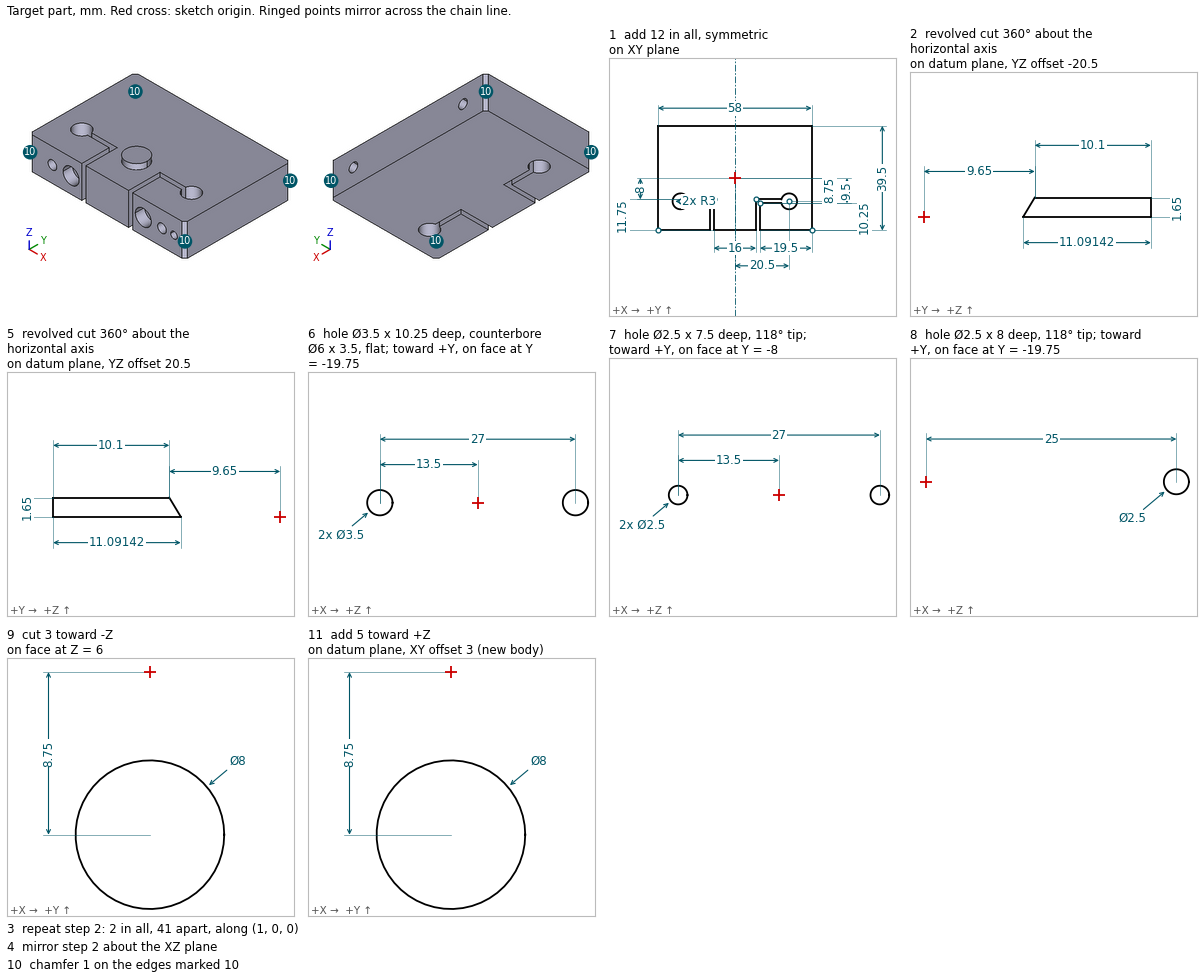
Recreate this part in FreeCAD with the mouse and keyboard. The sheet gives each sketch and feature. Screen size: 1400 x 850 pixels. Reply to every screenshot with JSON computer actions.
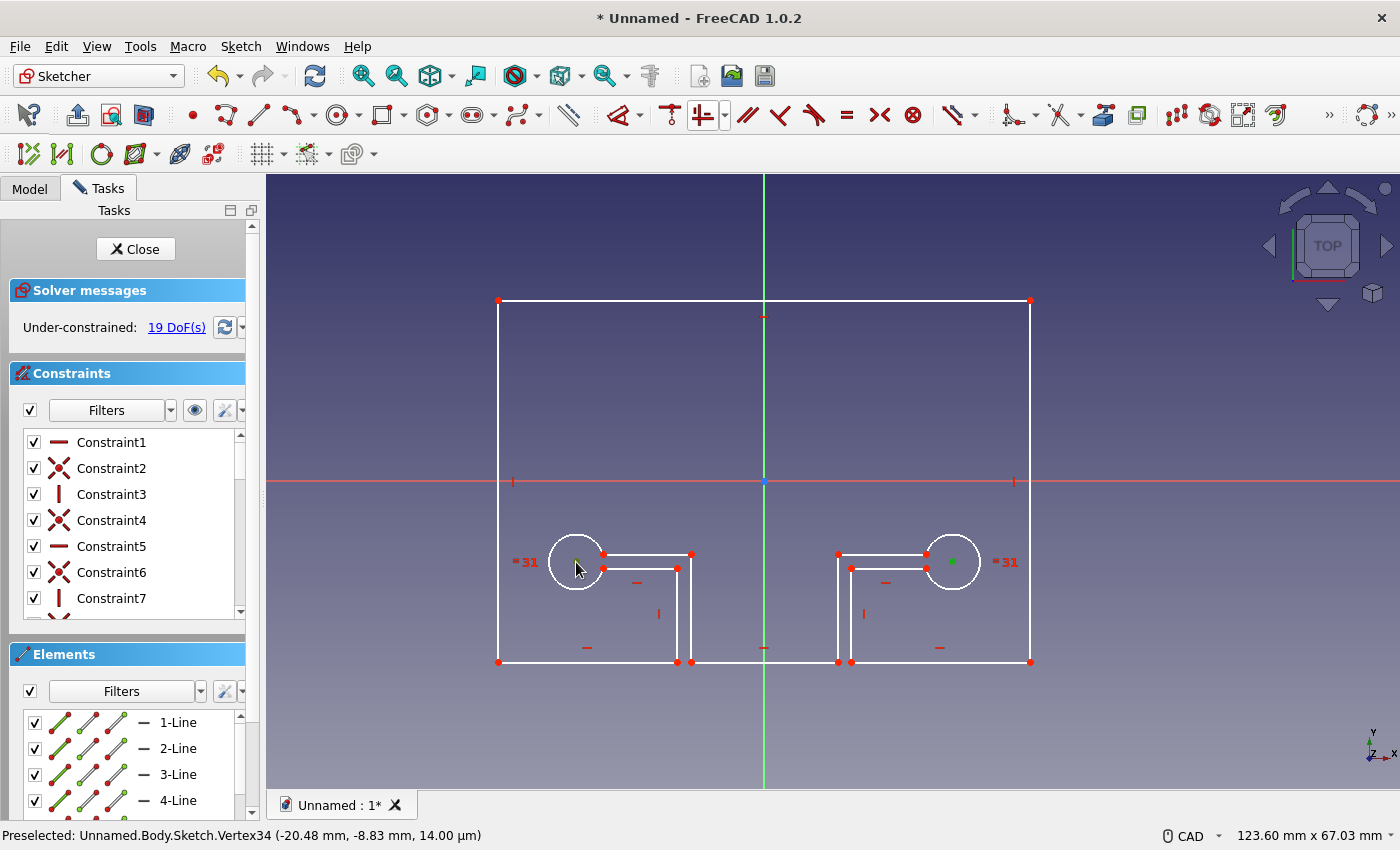
{"action": "left_click", "coordinate": [764, 721]}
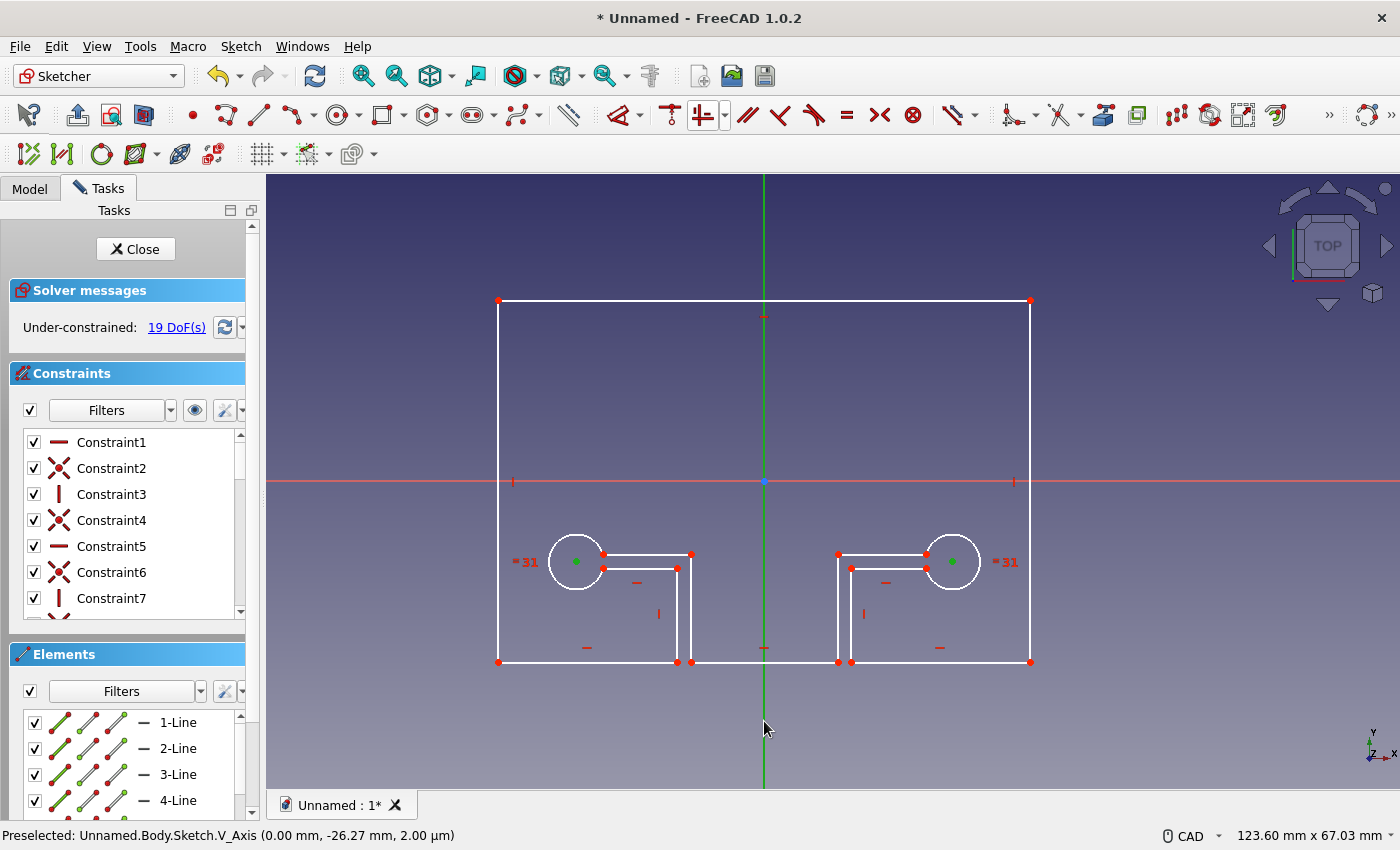
{"action": "left_click", "coordinate": [880, 116]}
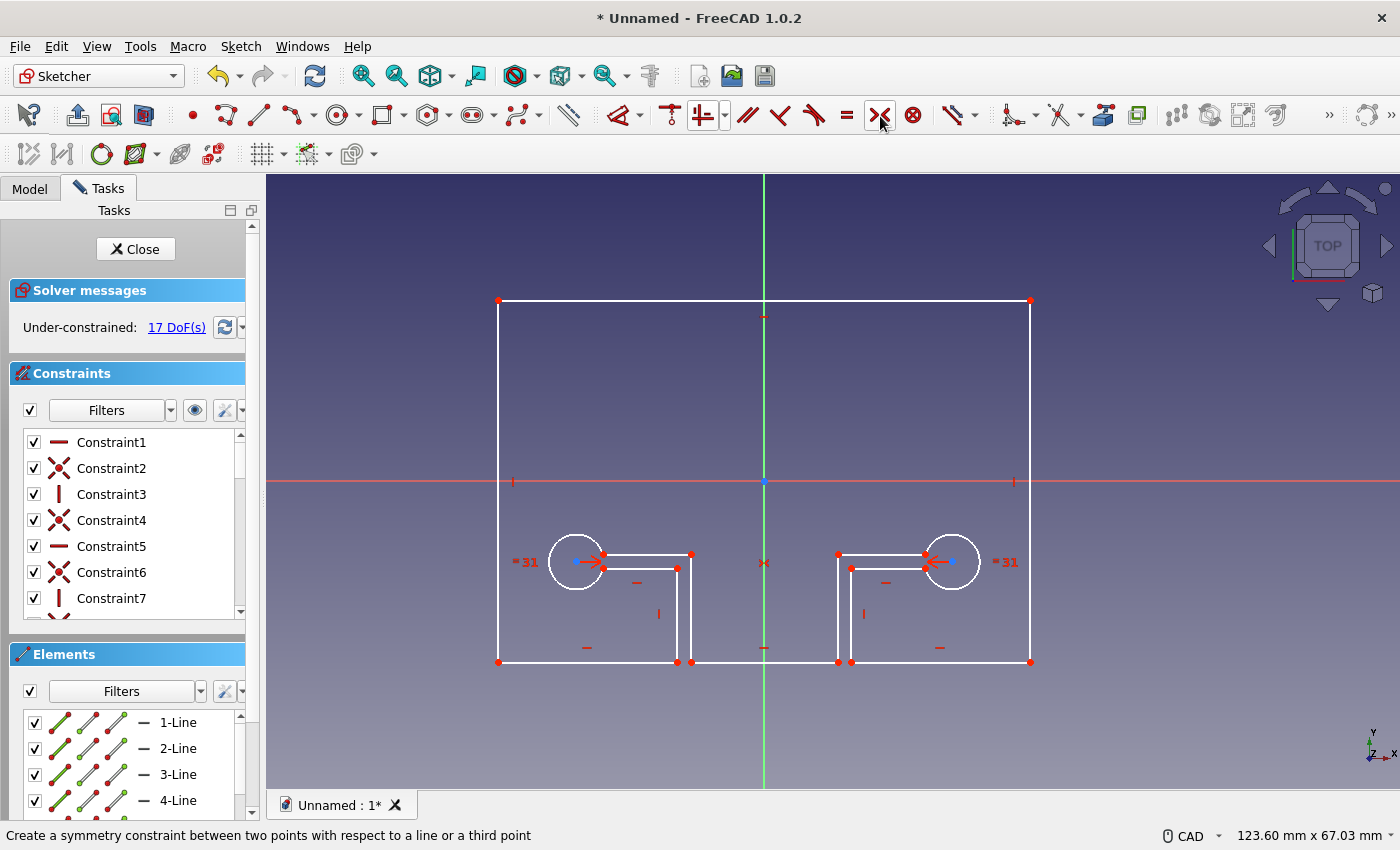
{"action": "left_click", "coordinate": [691, 555]}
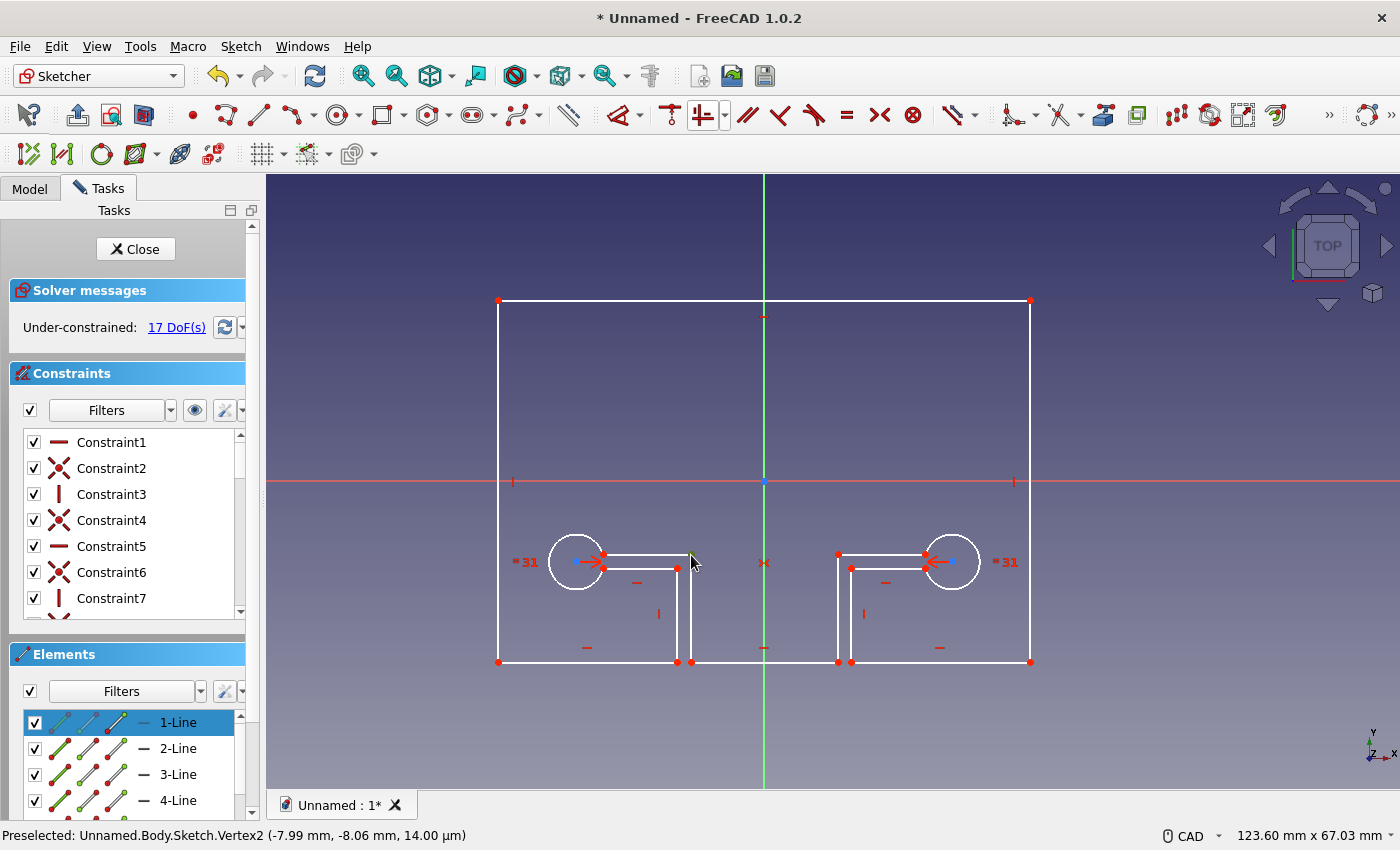
{"action": "left_click", "coordinate": [838, 555]}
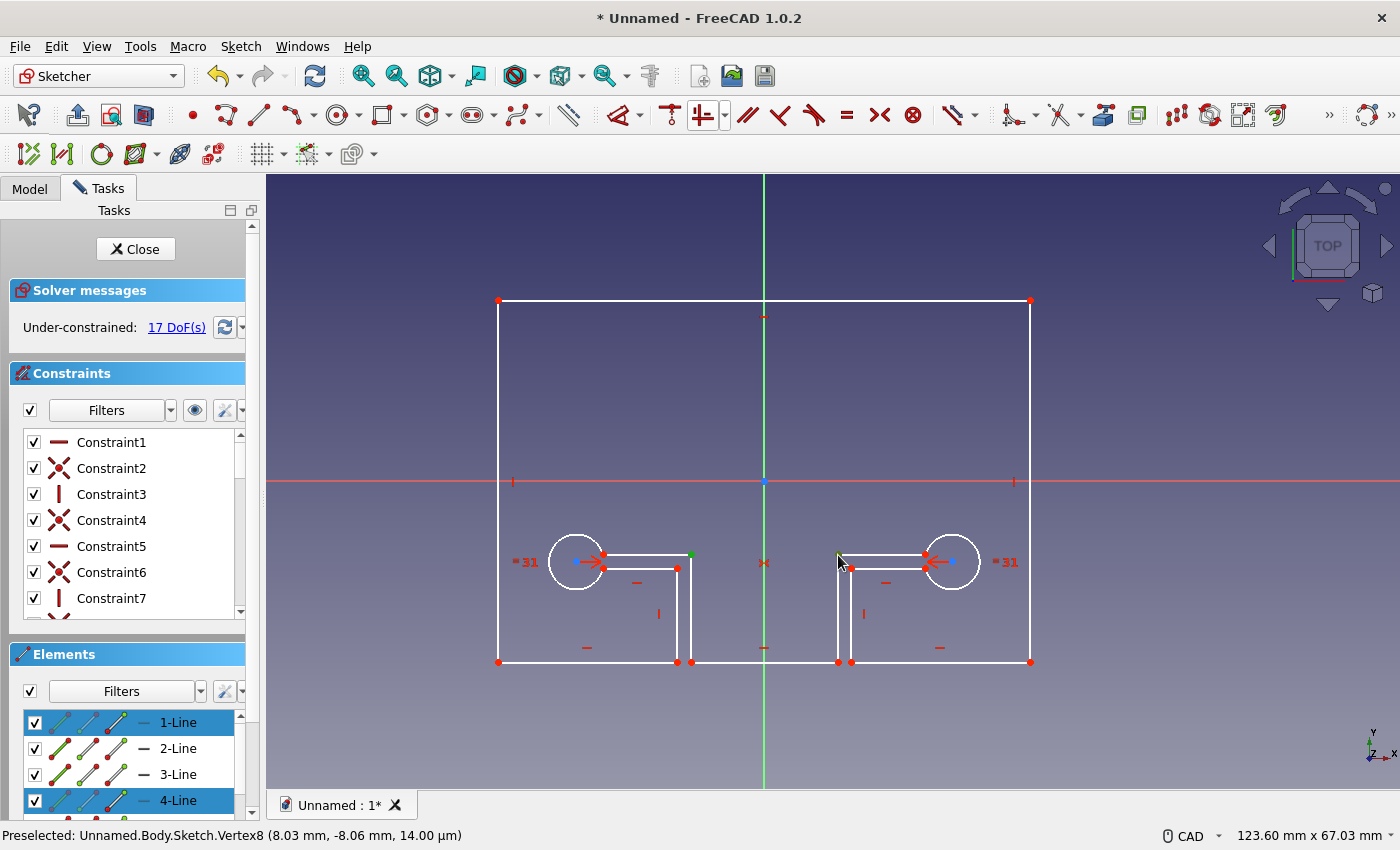
{"action": "left_click", "coordinate": [764, 721]}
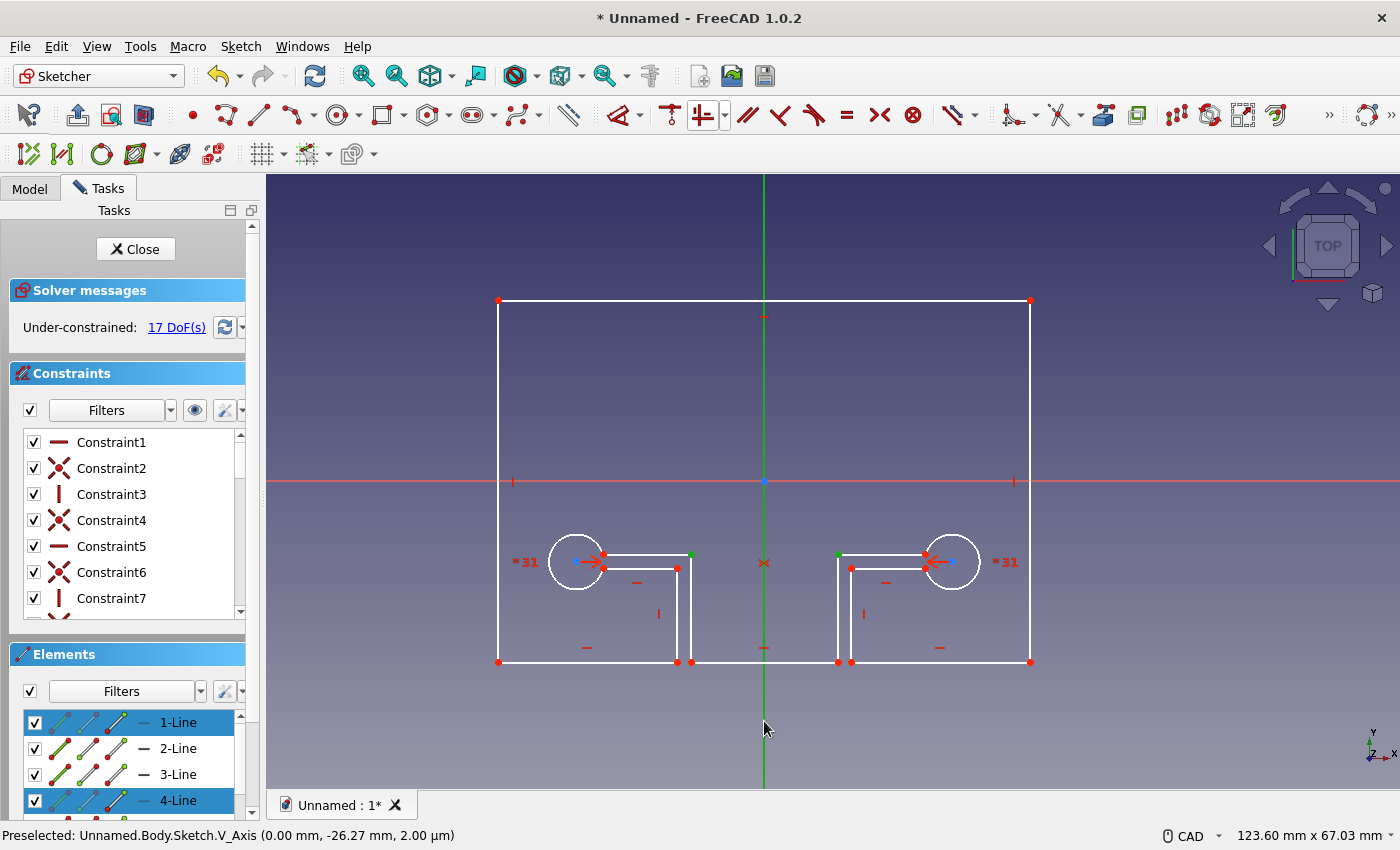
{"action": "left_click", "coordinate": [880, 116]}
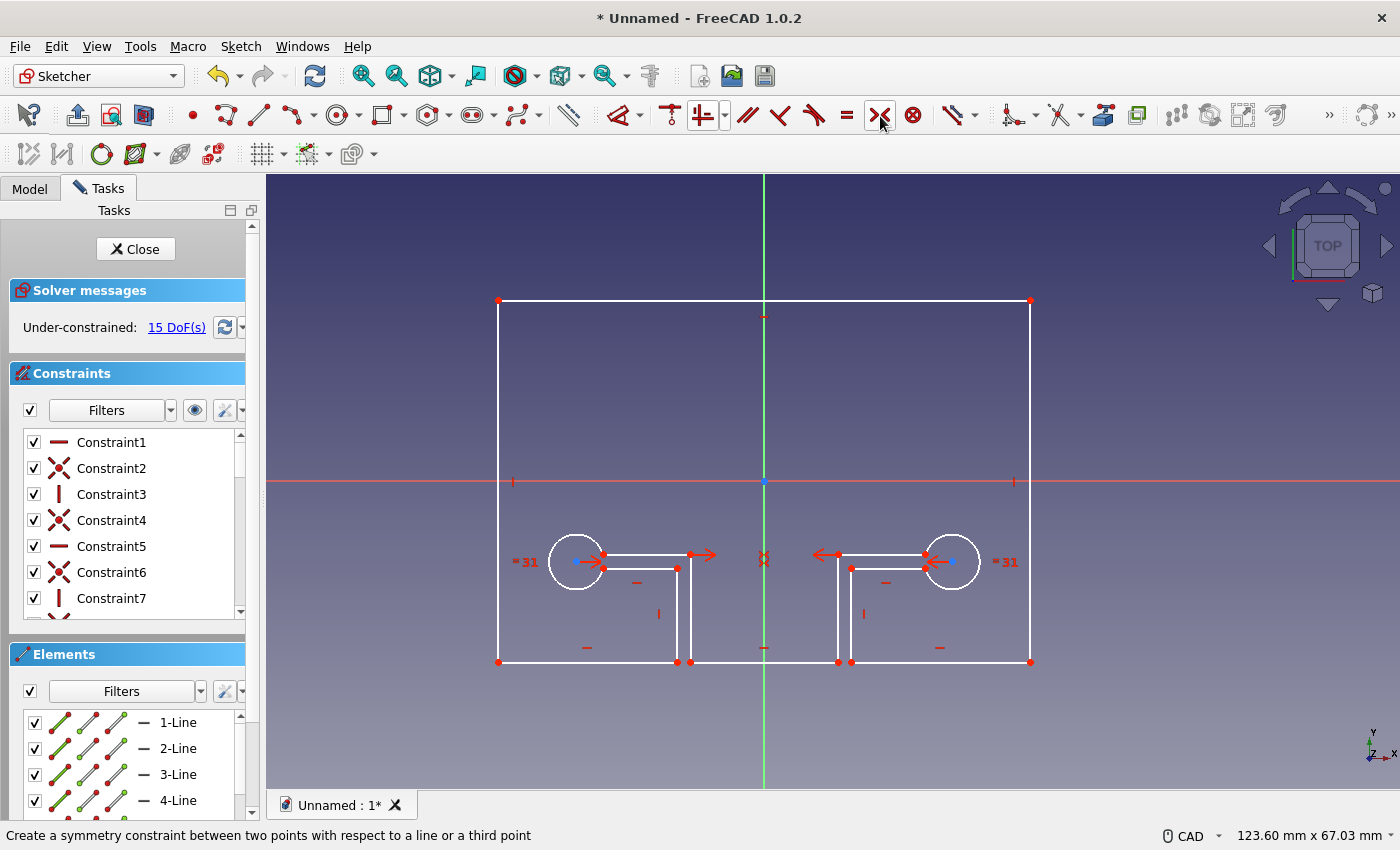
{"action": "left_click", "coordinate": [1030, 663]}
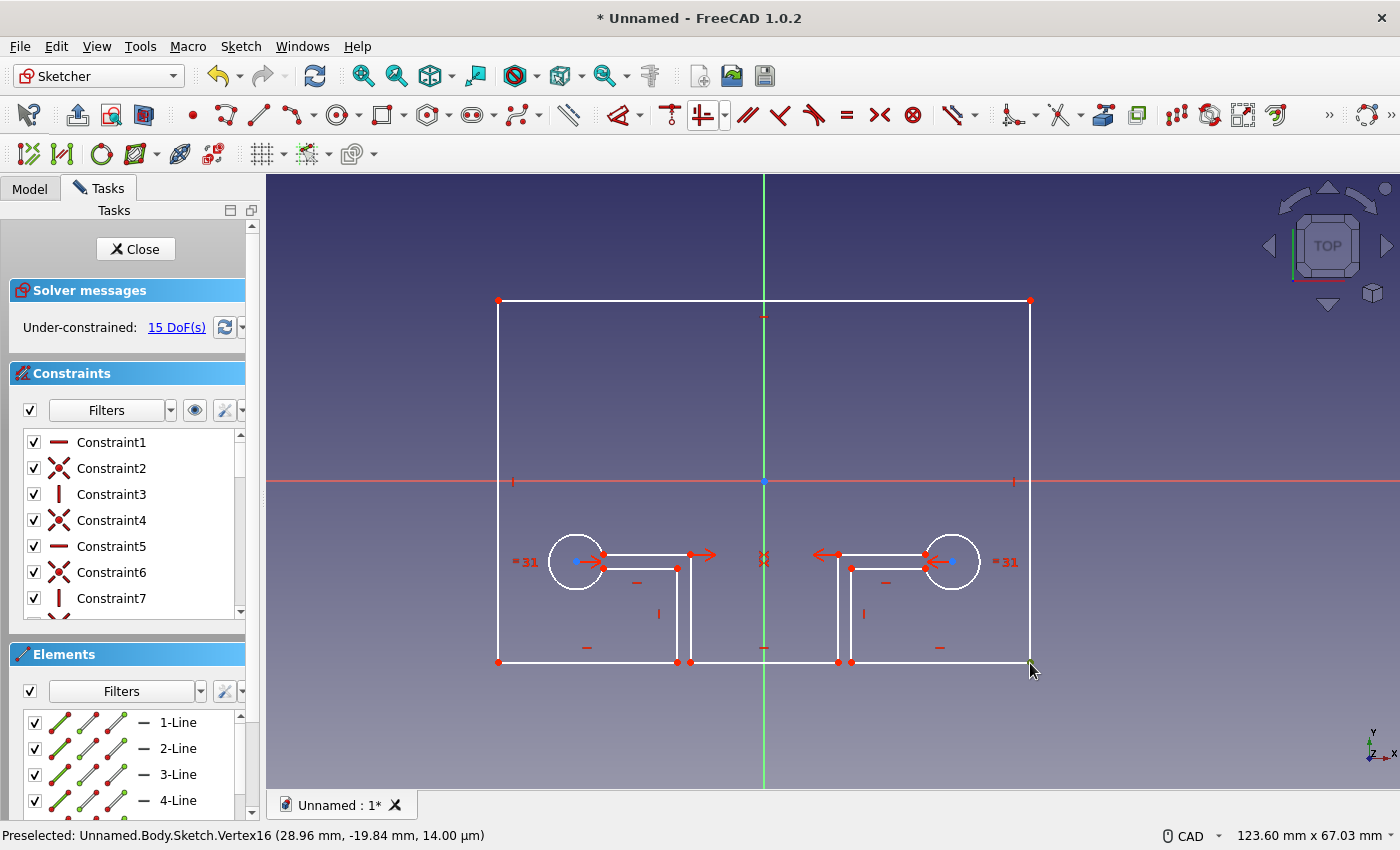
{"action": "left_click", "coordinate": [498, 663]}